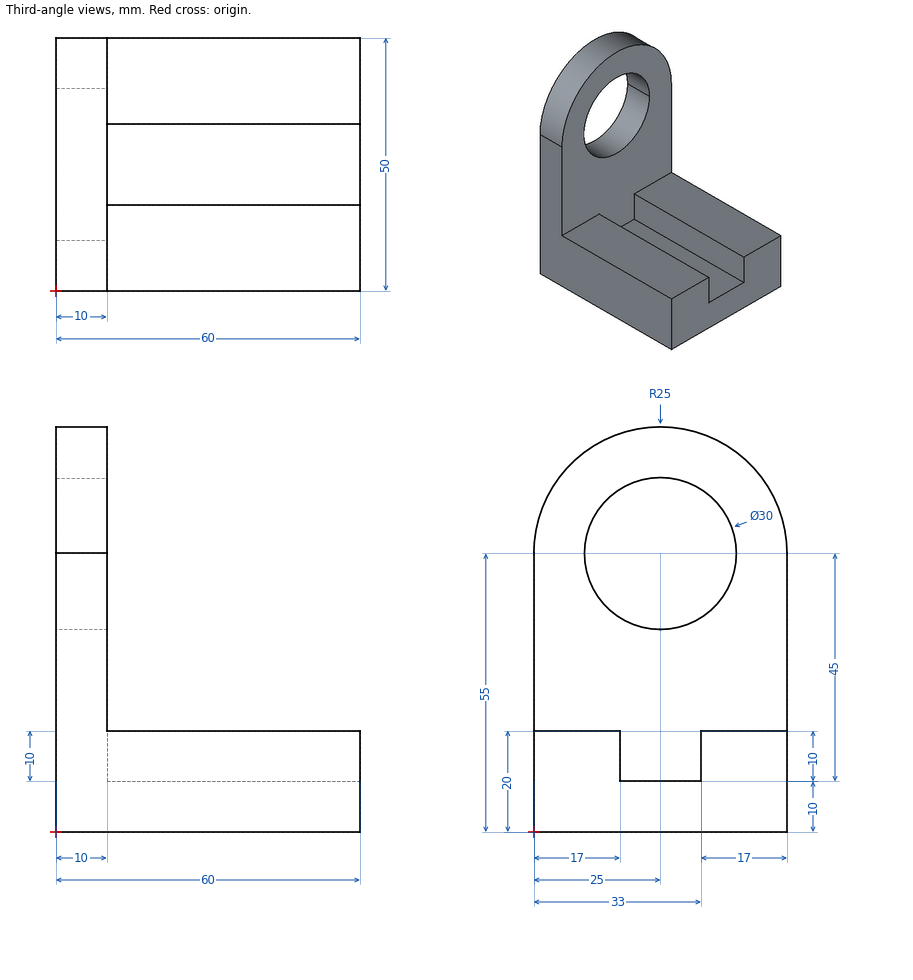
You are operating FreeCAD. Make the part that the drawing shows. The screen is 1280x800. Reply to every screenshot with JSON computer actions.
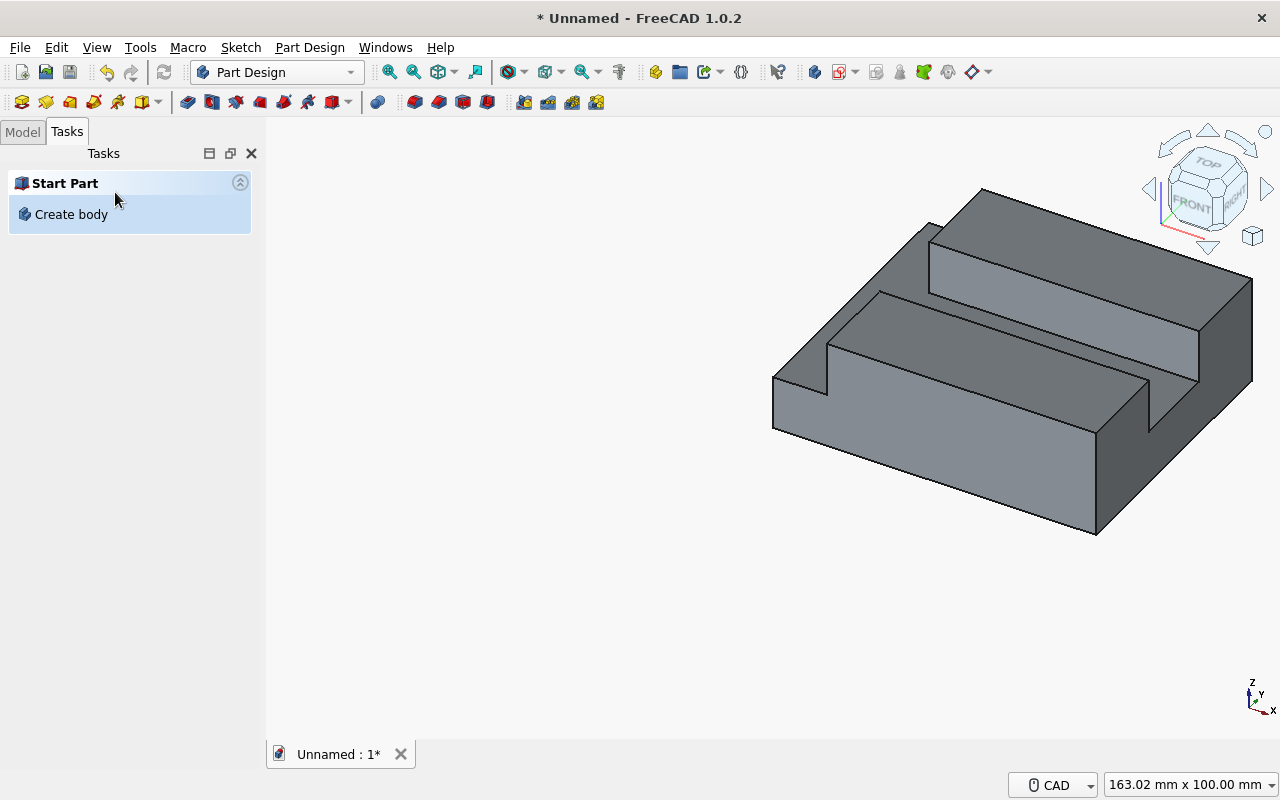
{"action": "left_click", "coordinate": [840, 72]}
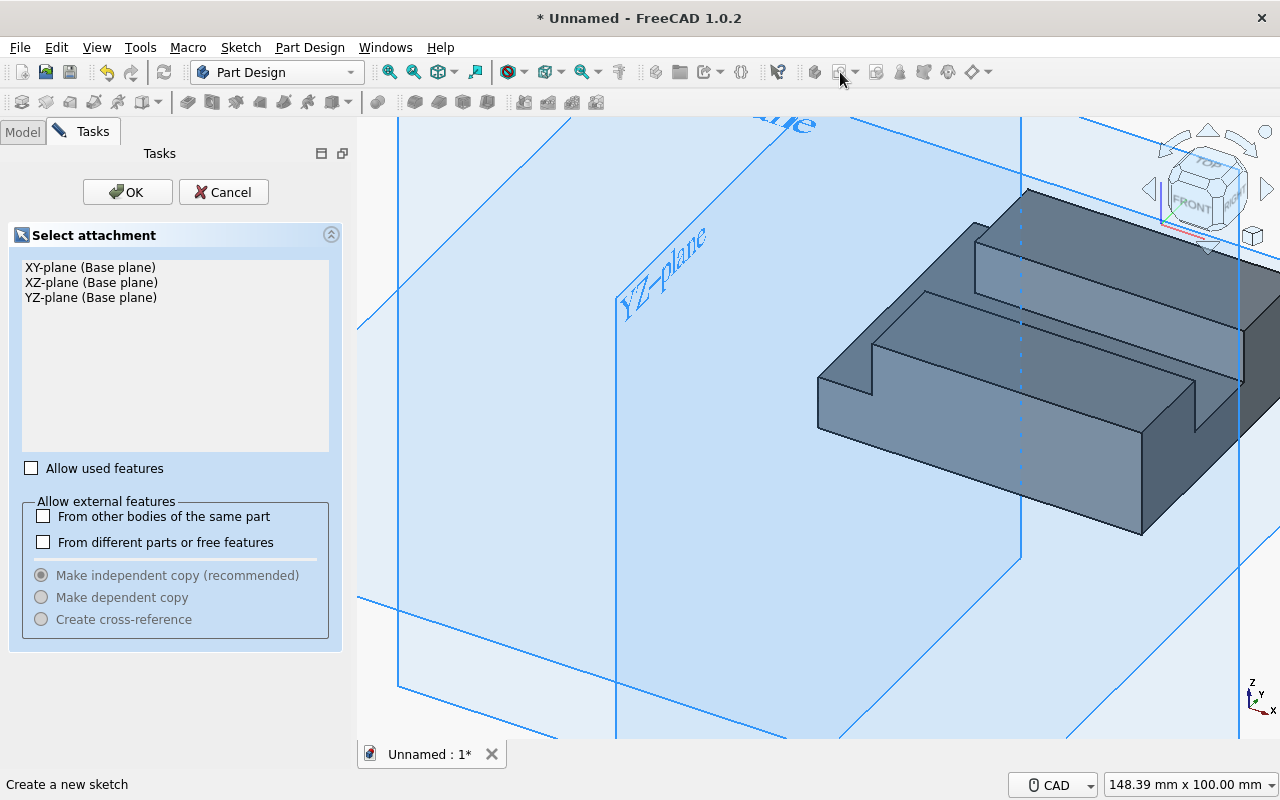
{"action": "left_click", "coordinate": [82, 298]}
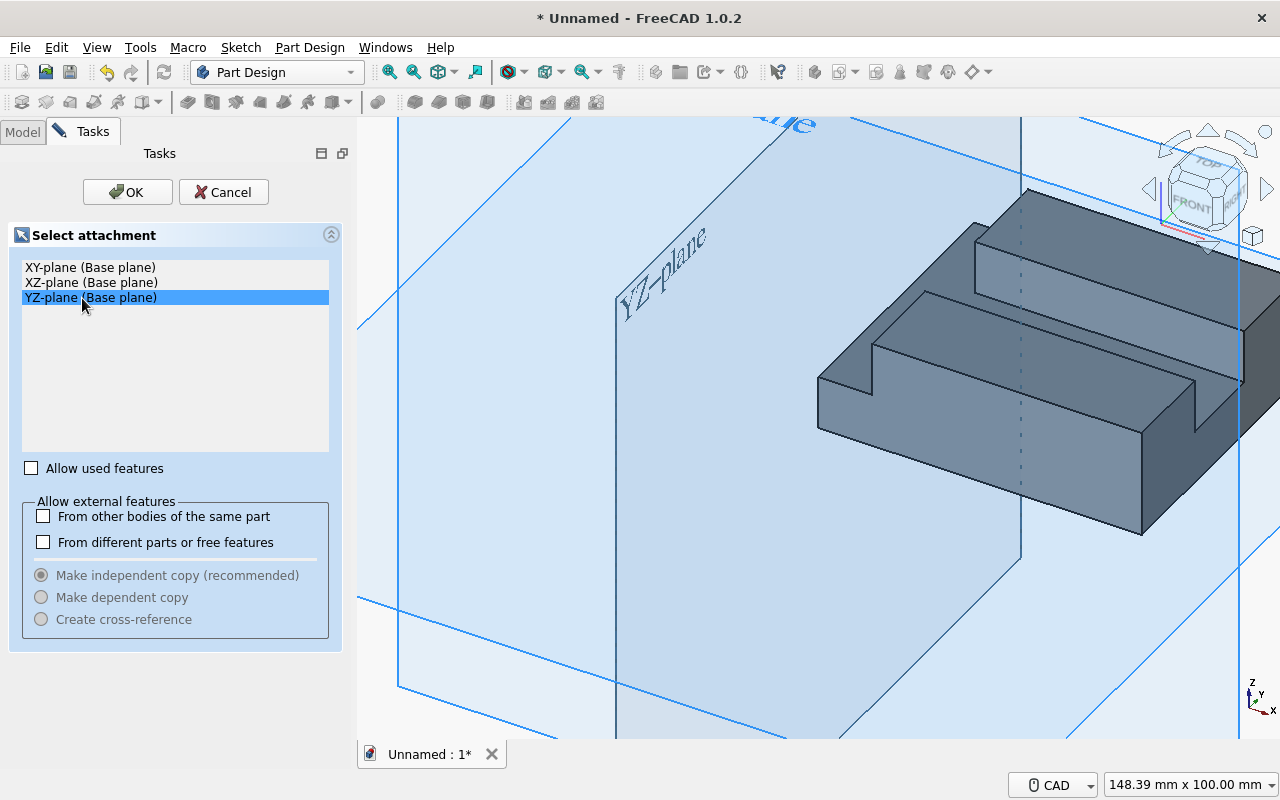
{"action": "left_click", "coordinate": [128, 192]}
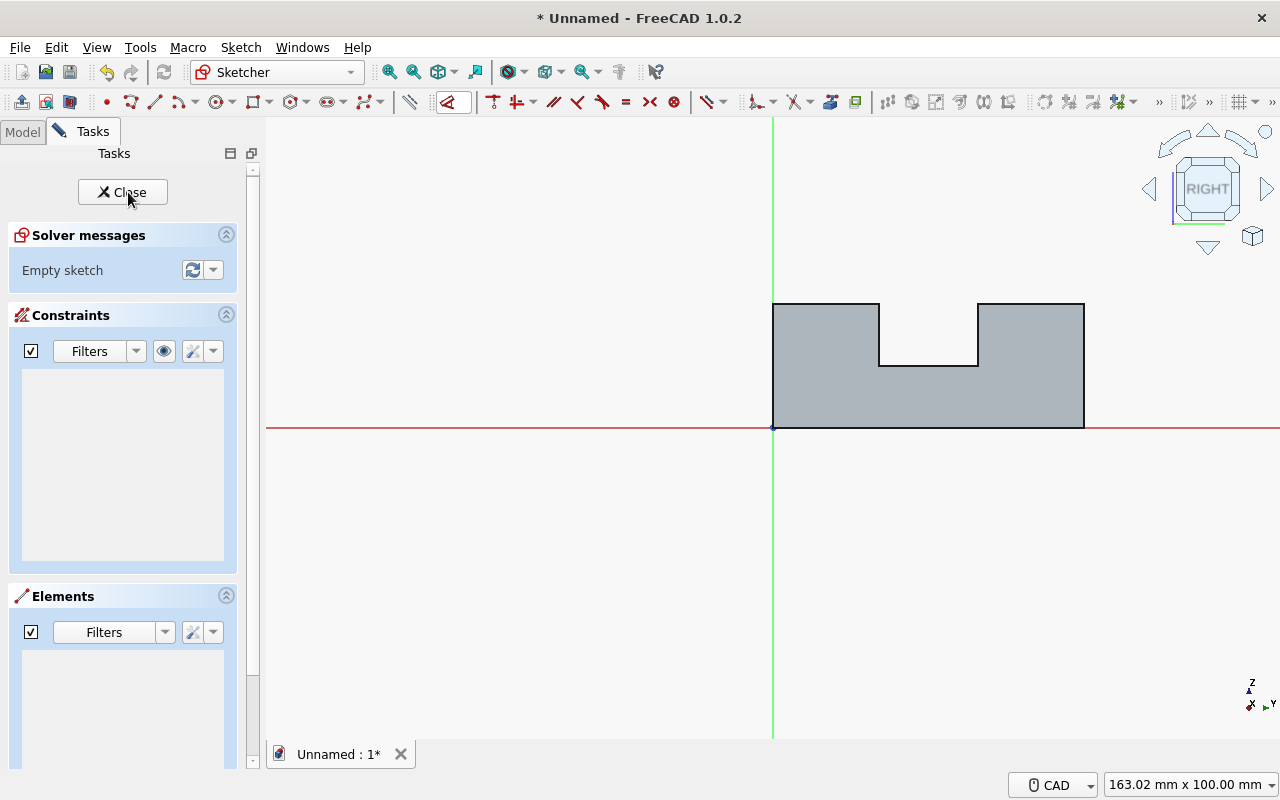
{"action": "left_click", "coordinate": [70, 102]}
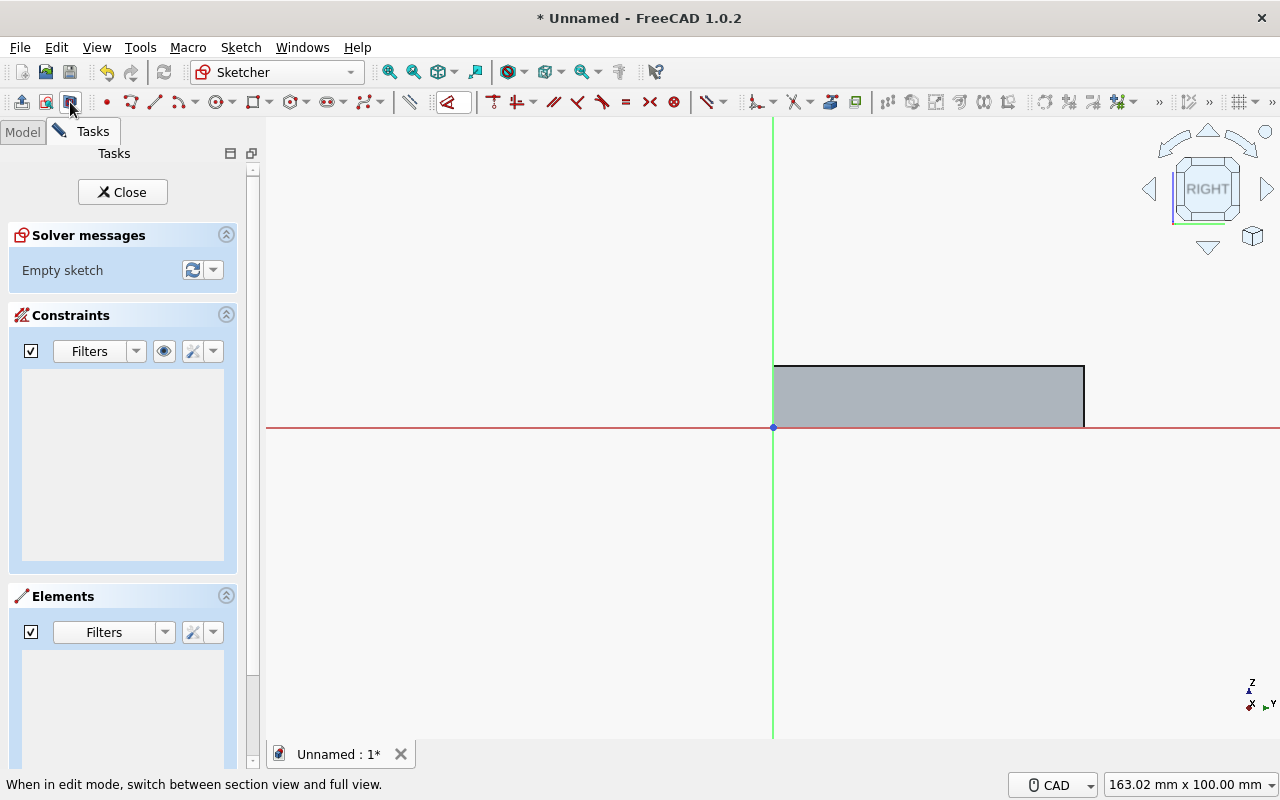
{"action": "scroll", "coordinate": [294, 711], "scroll_direction": "down", "scroll_amount": 2}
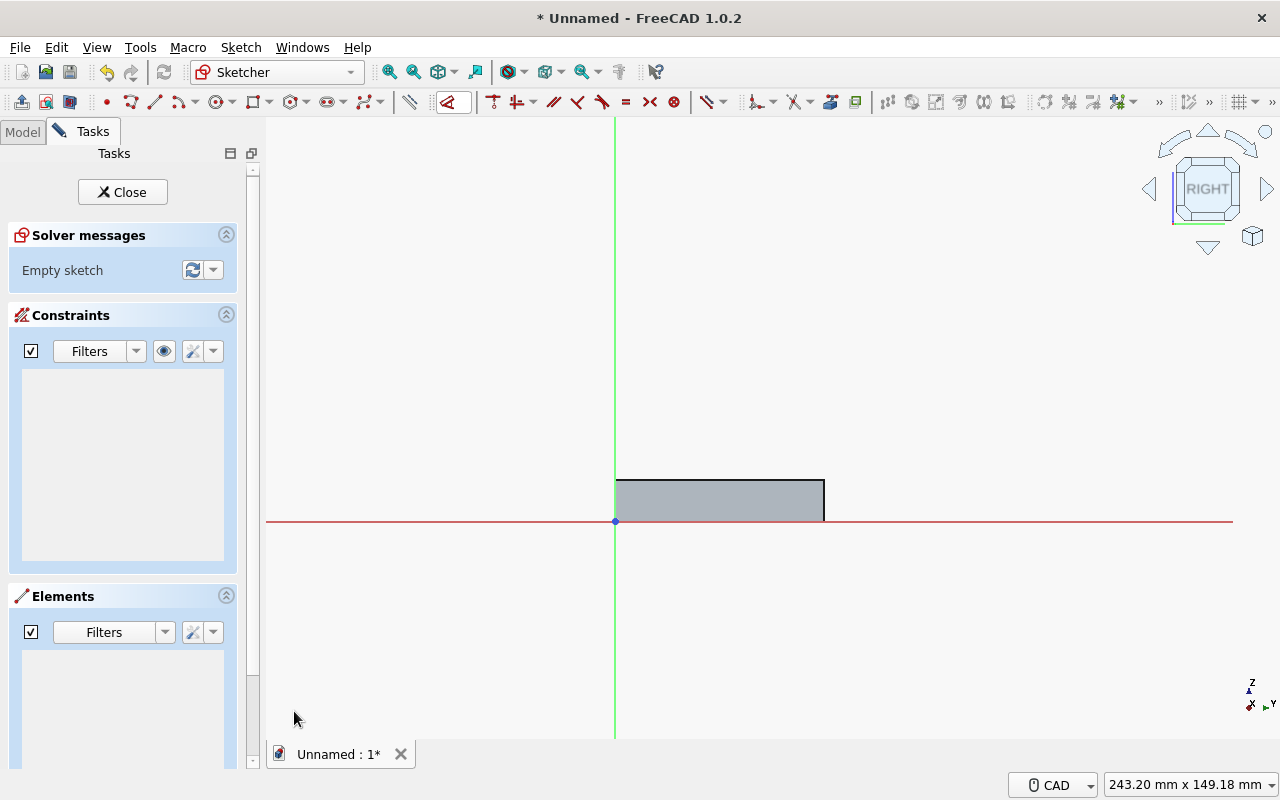
{"action": "left_click", "coordinate": [132, 102]}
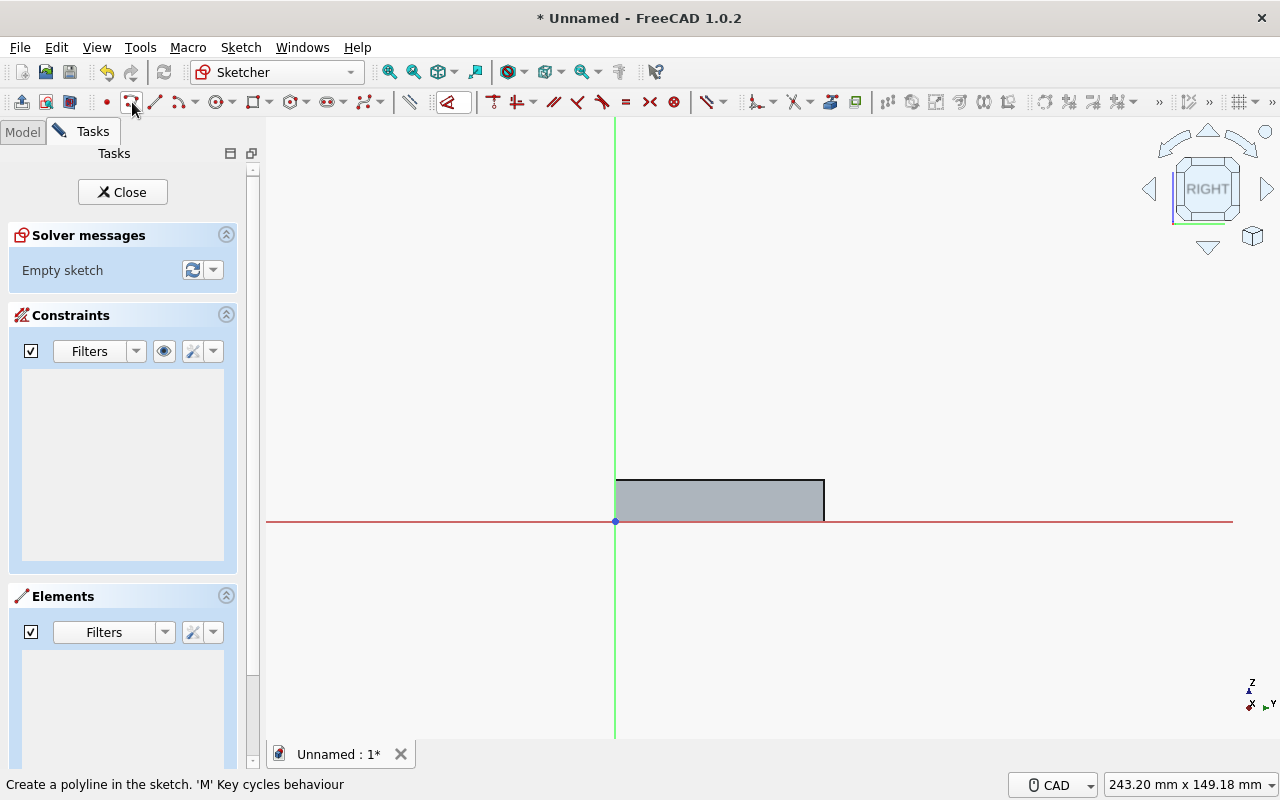
{"action": "left_click", "coordinate": [824, 292]}
{"action": "left_click", "coordinate": [824, 480]}
{"action": "left_click", "coordinate": [615, 480]}
{"action": "left_click", "coordinate": [624, 292]}
{"action": "right_click", "coordinate": [624, 292]}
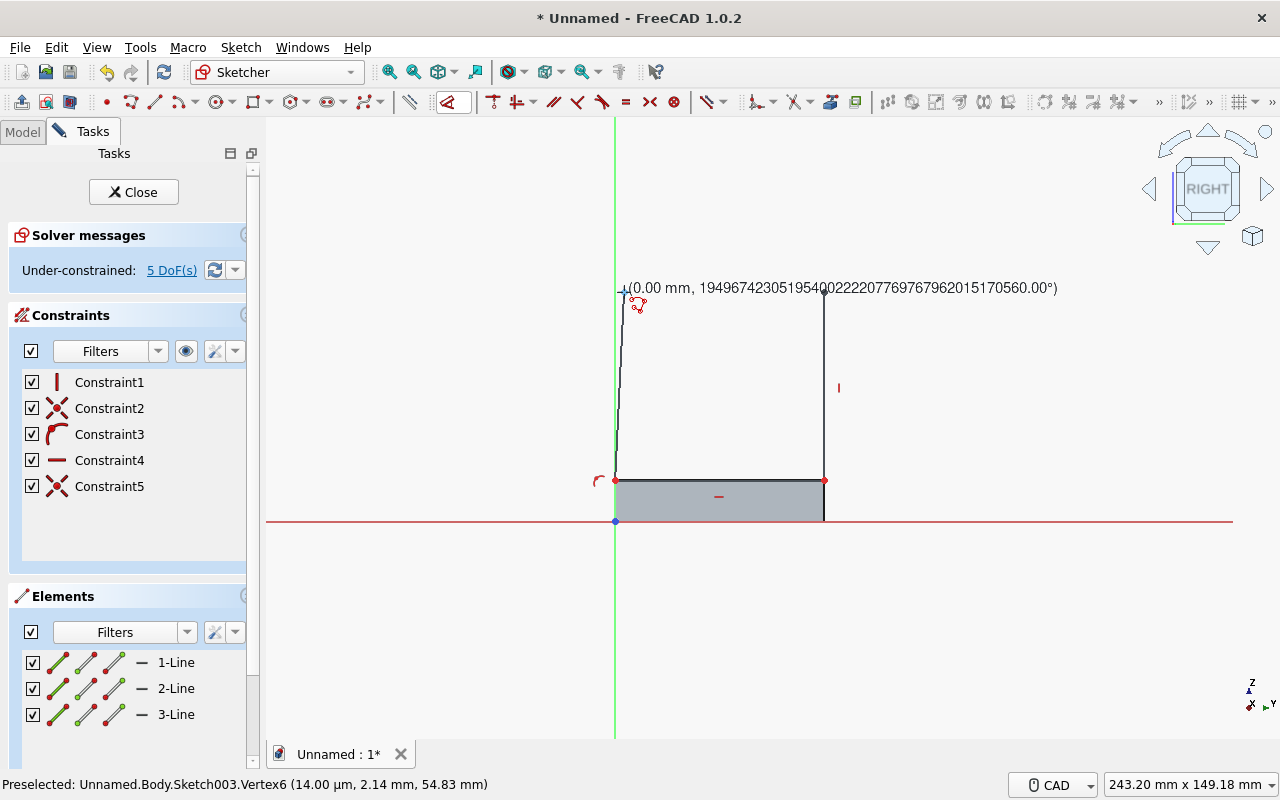
{"action": "left_click", "coordinate": [198, 102]}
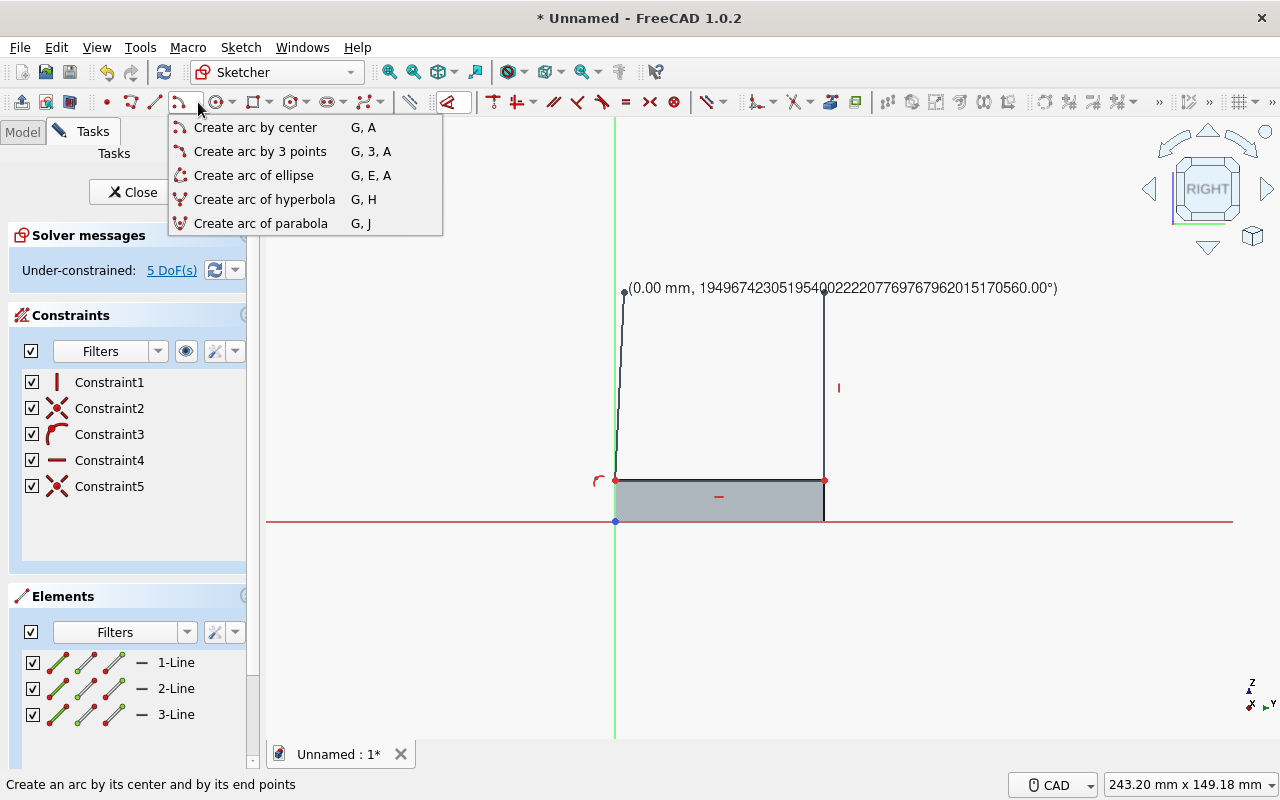
{"action": "left_click", "coordinate": [306, 151]}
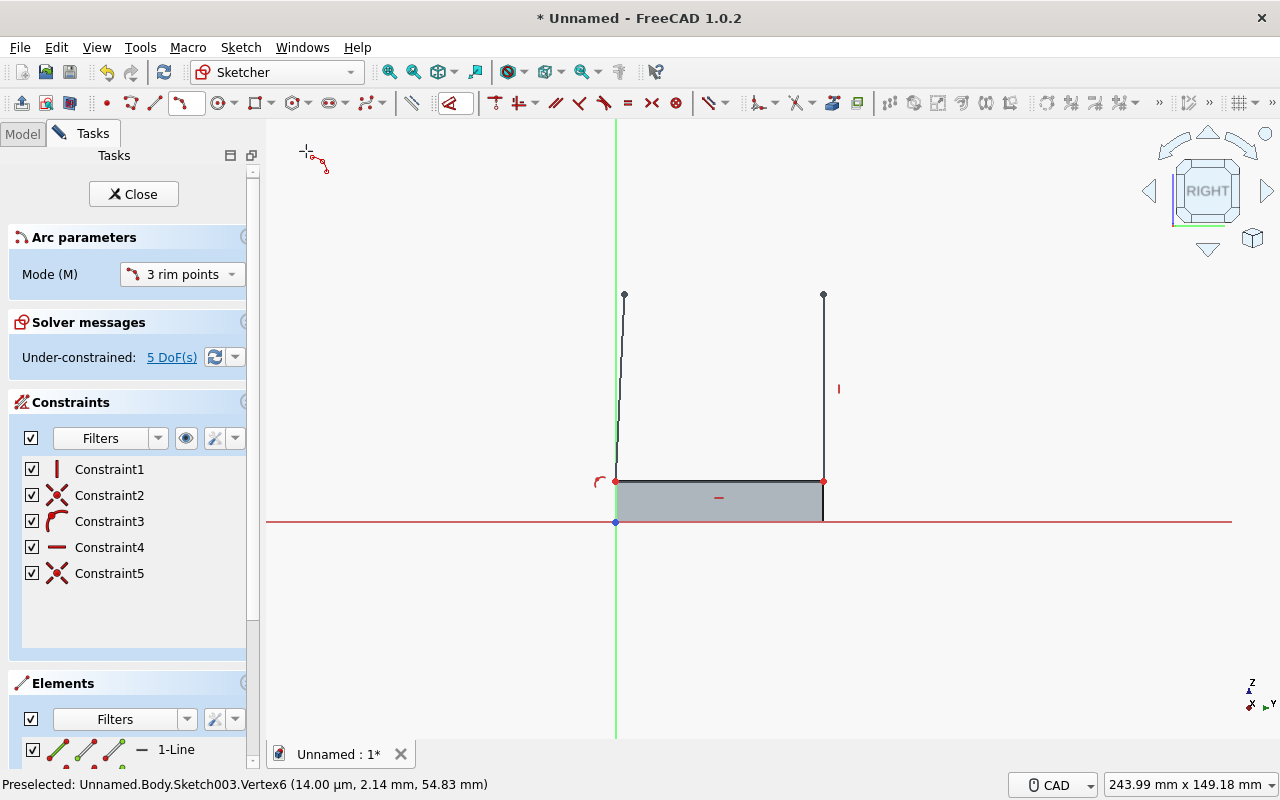
{"action": "left_click", "coordinate": [624, 294]}
{"action": "left_click", "coordinate": [824, 294]}
{"action": "left_click", "coordinate": [719, 190]}
{"action": "key", "text": "Escape"}